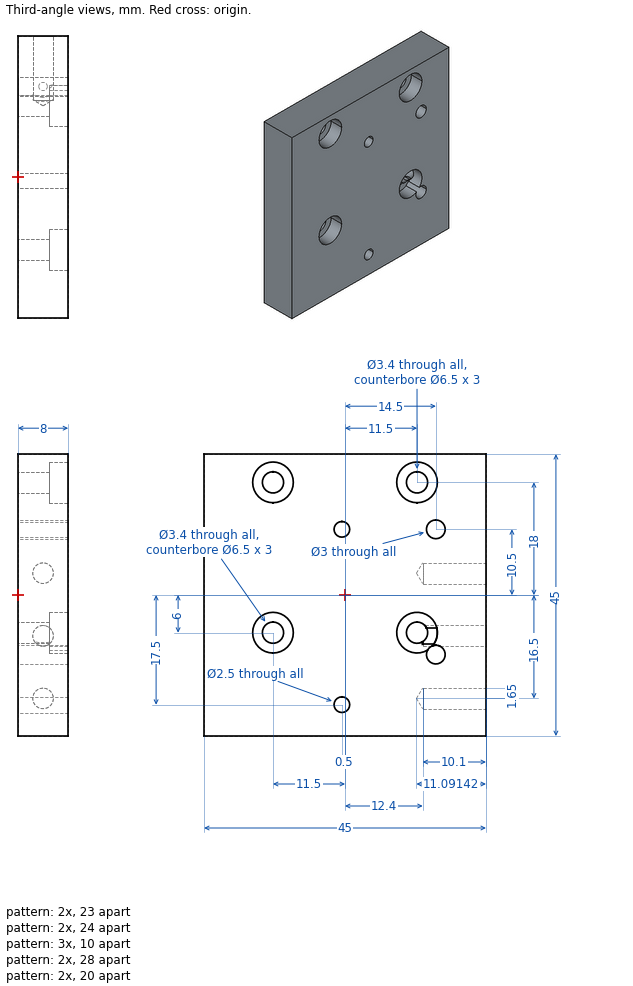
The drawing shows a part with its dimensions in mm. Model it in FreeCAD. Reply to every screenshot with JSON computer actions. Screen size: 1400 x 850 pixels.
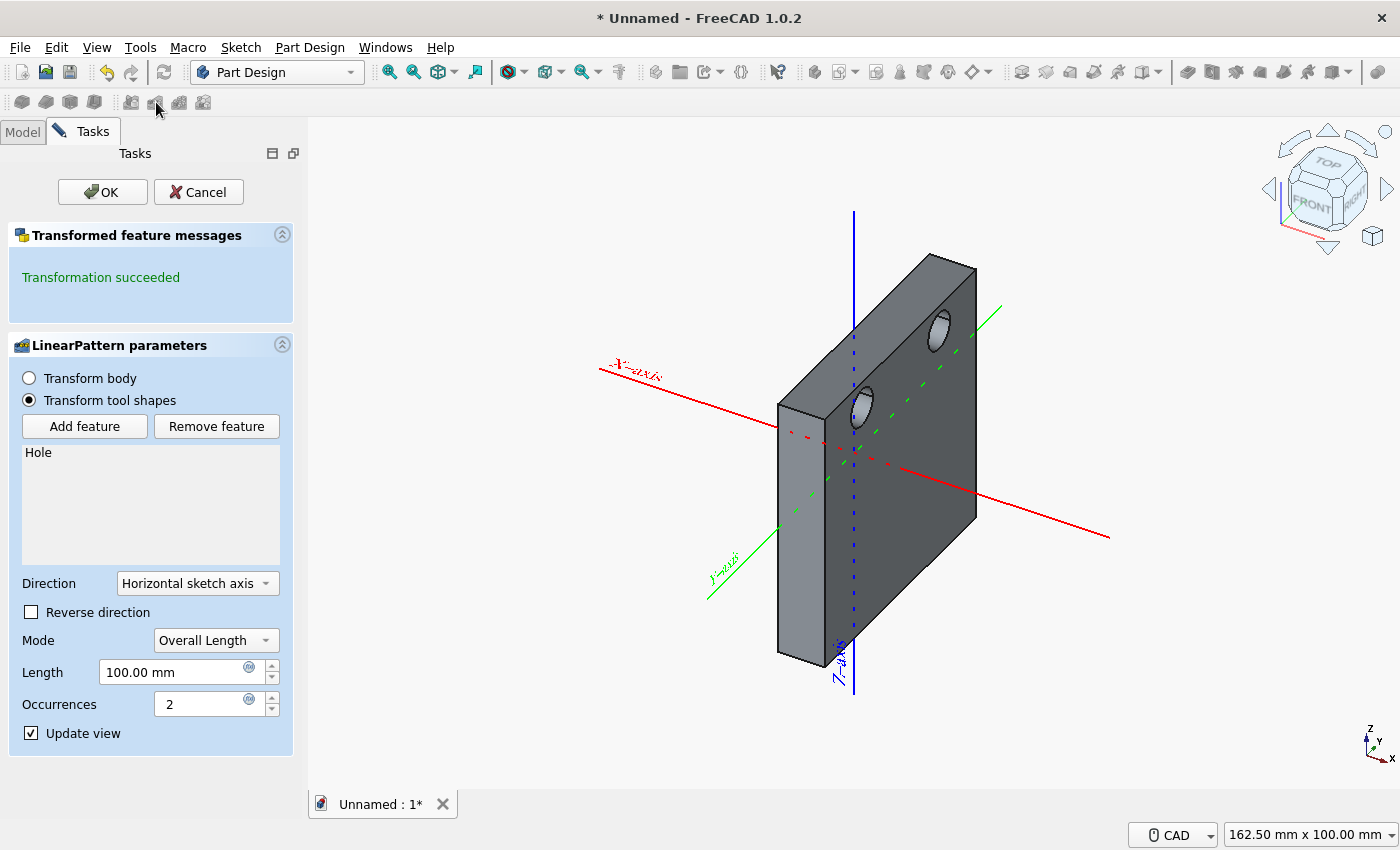
{"action": "left_click", "coordinate": [198, 584]}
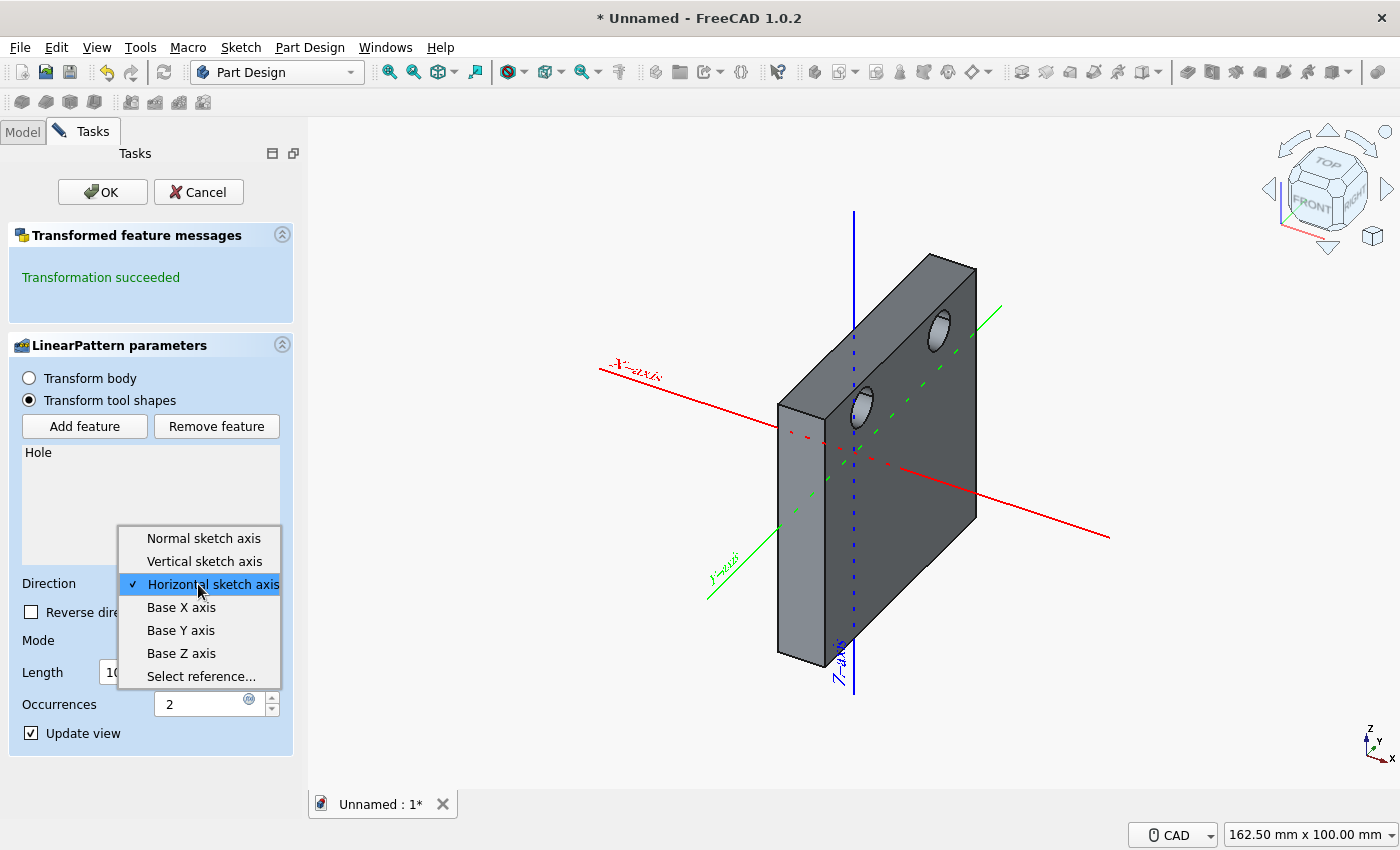
{"action": "left_click", "coordinate": [198, 654]}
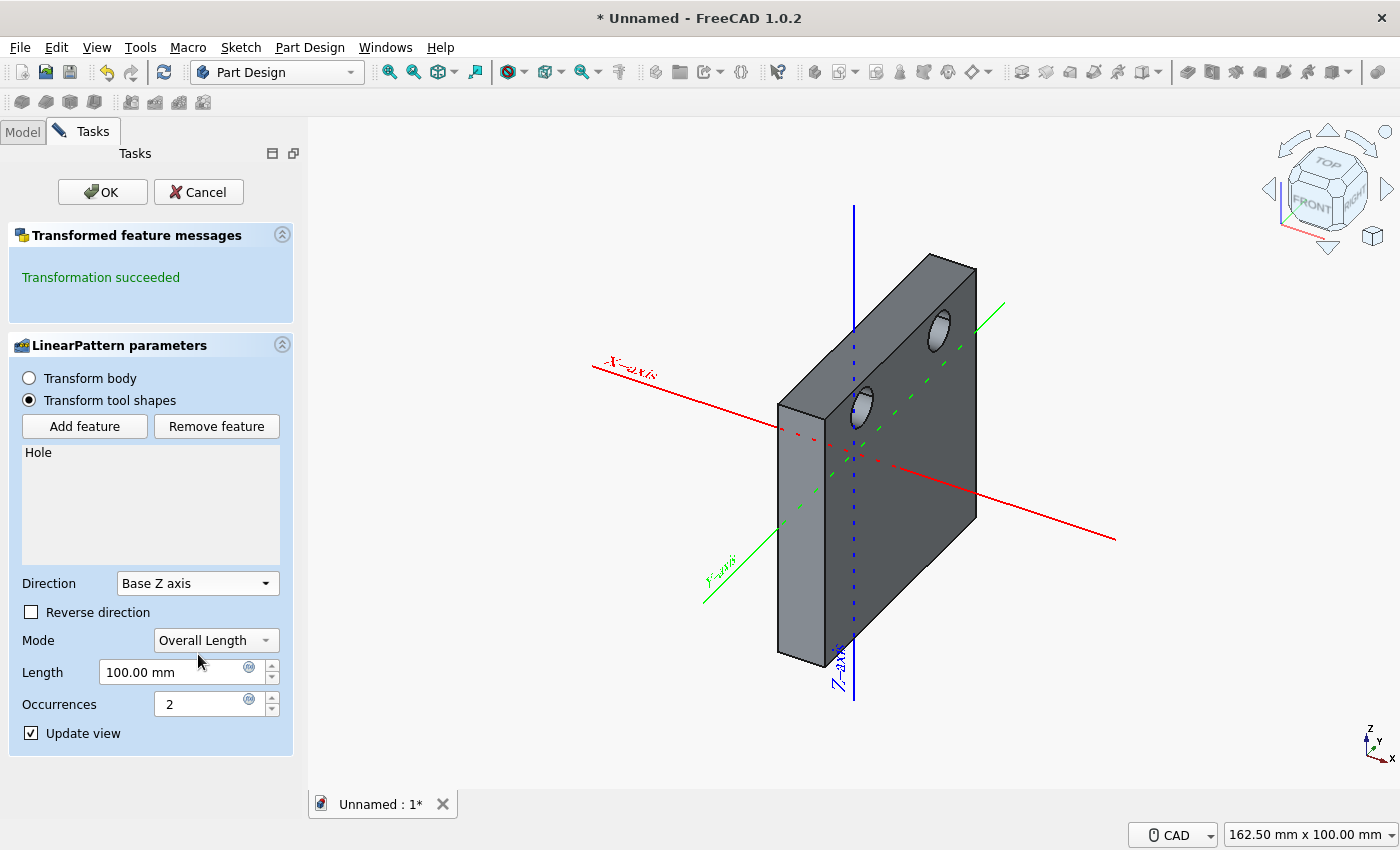
{"action": "left_click", "coordinate": [217, 640]}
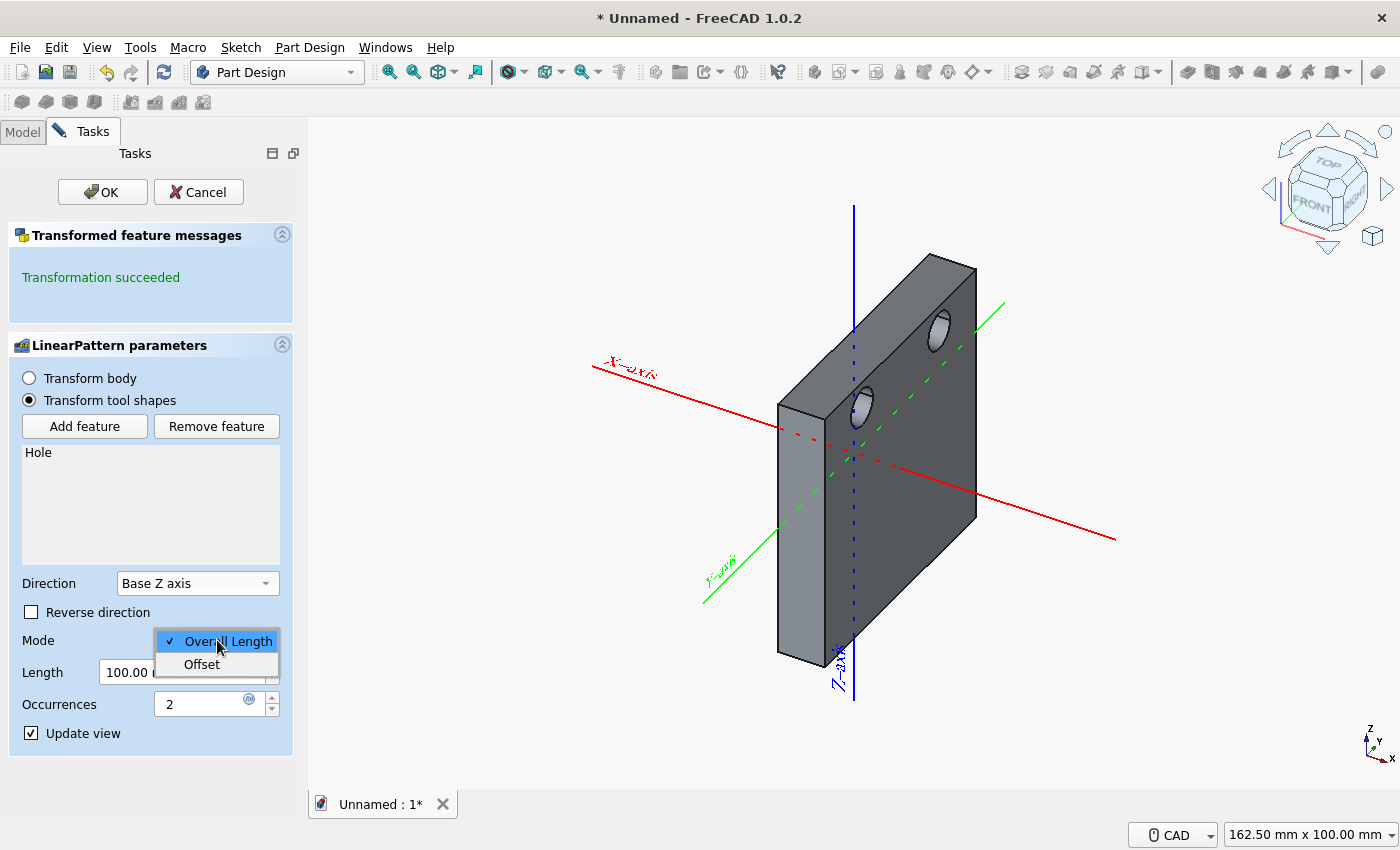
{"action": "left_click", "coordinate": [216, 664]}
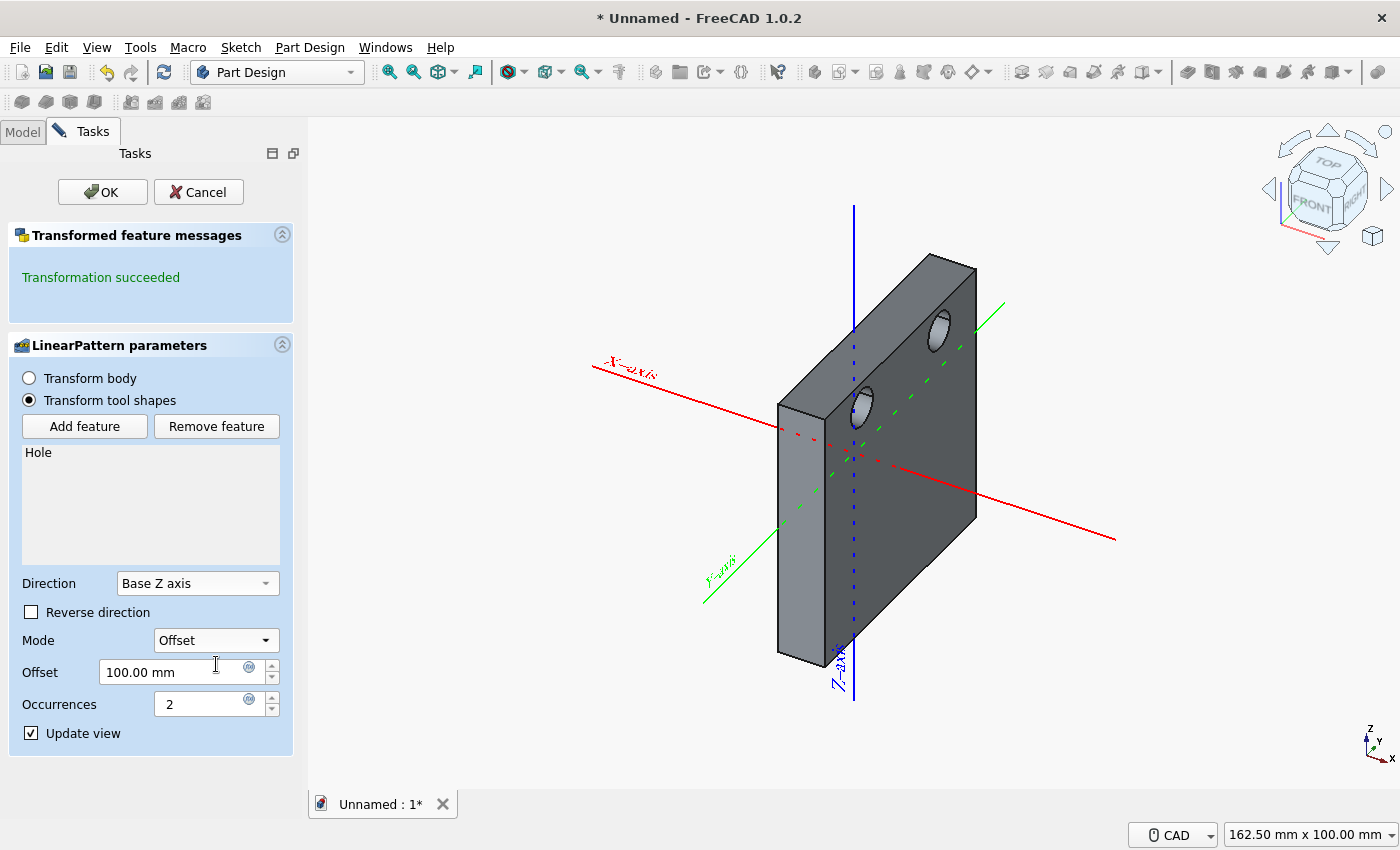
{"action": "triple_click", "coordinate": [182, 672]}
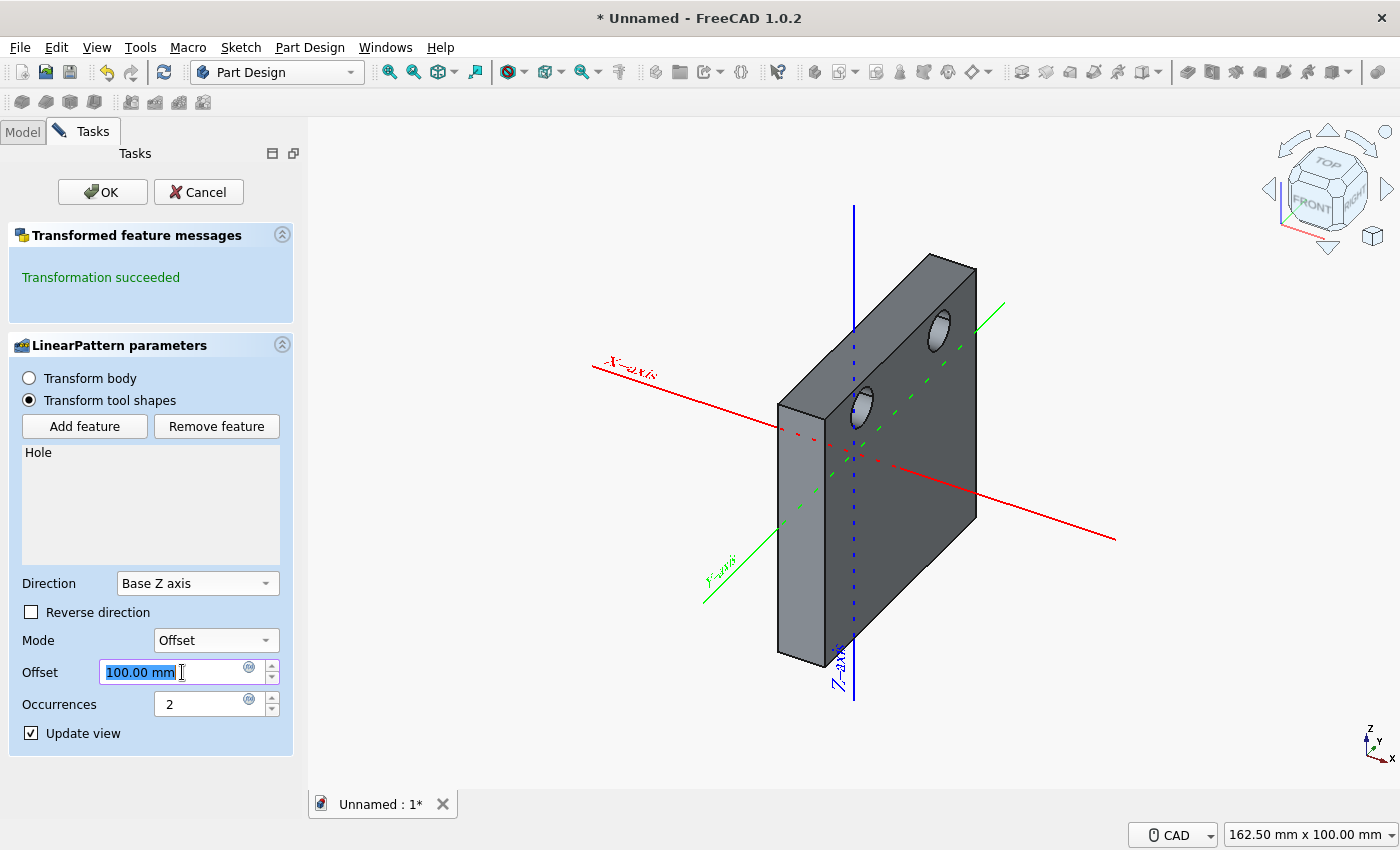
{"action": "type", "text": "24"}
{"action": "key", "text": "Tab"}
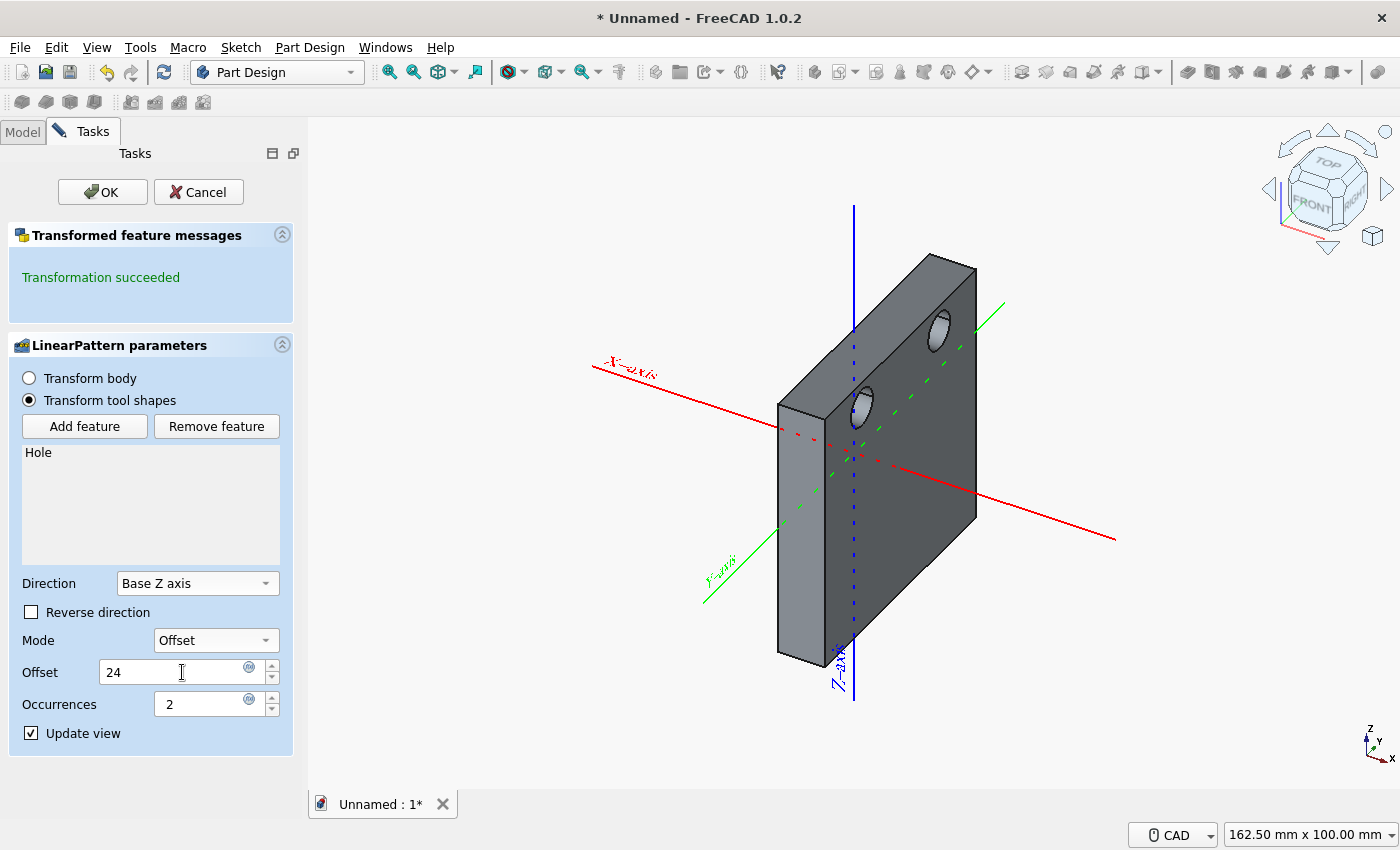
{"action": "triple_click", "coordinate": [209, 704]}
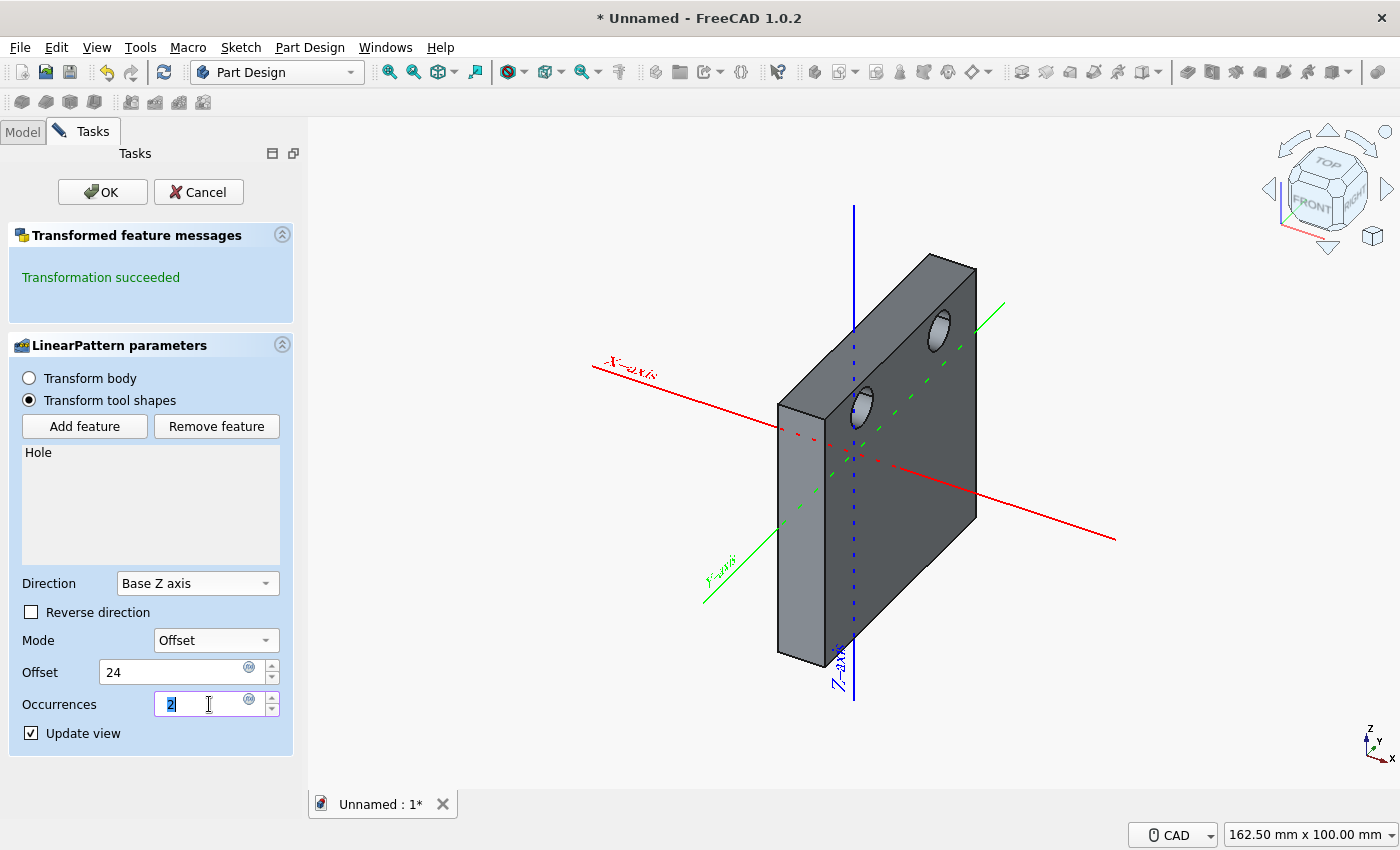
{"action": "type", "text": "2"}
{"action": "key", "text": "Tab"}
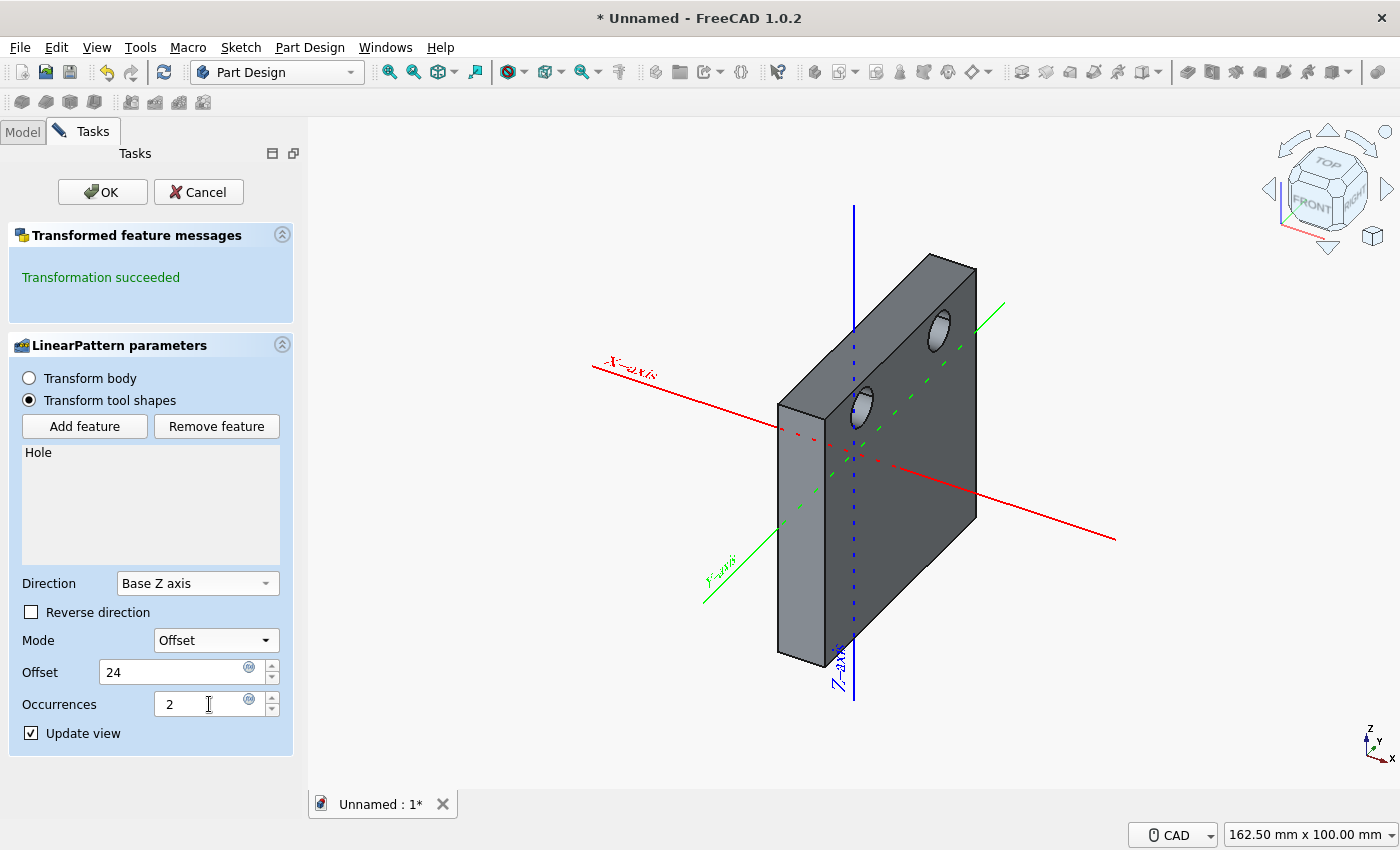
{"action": "left_click", "coordinate": [30, 612]}